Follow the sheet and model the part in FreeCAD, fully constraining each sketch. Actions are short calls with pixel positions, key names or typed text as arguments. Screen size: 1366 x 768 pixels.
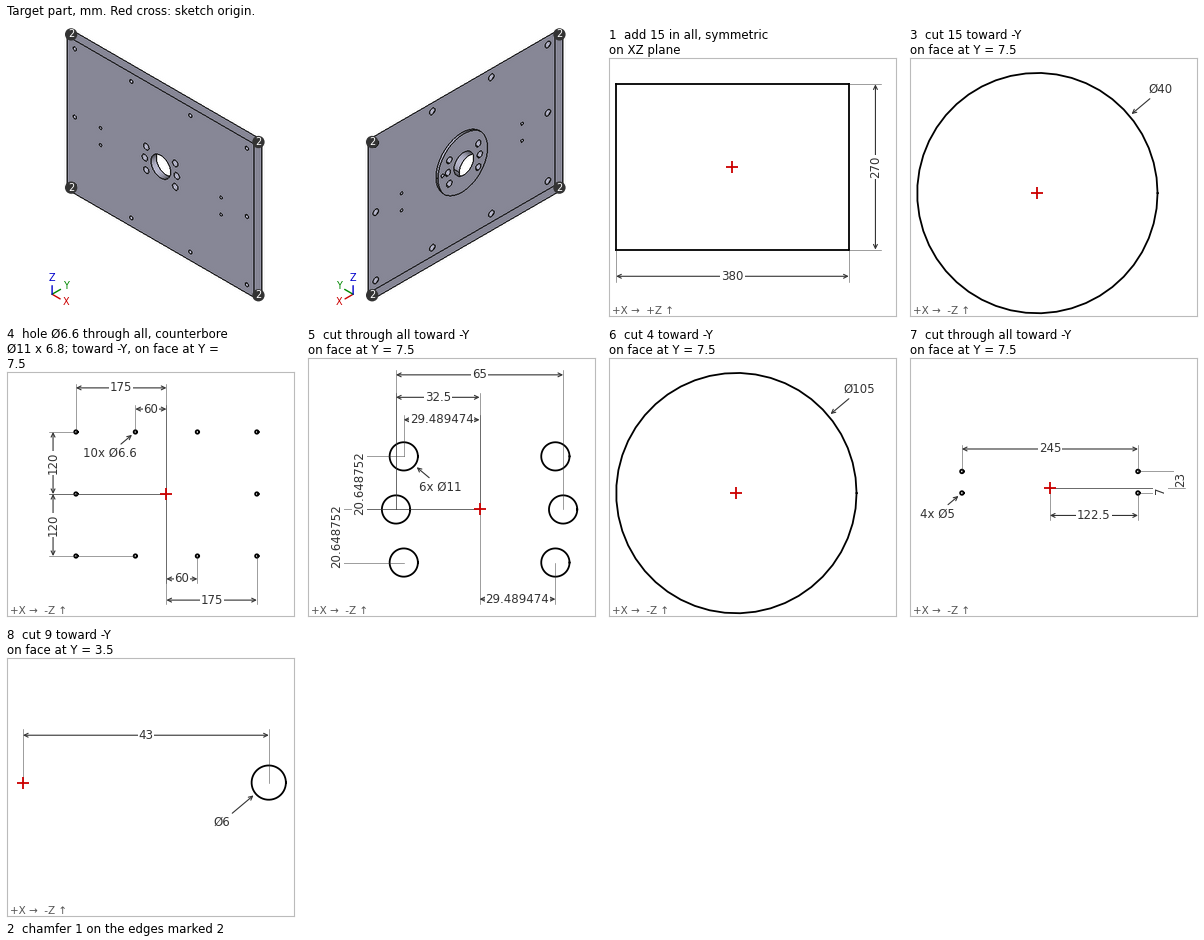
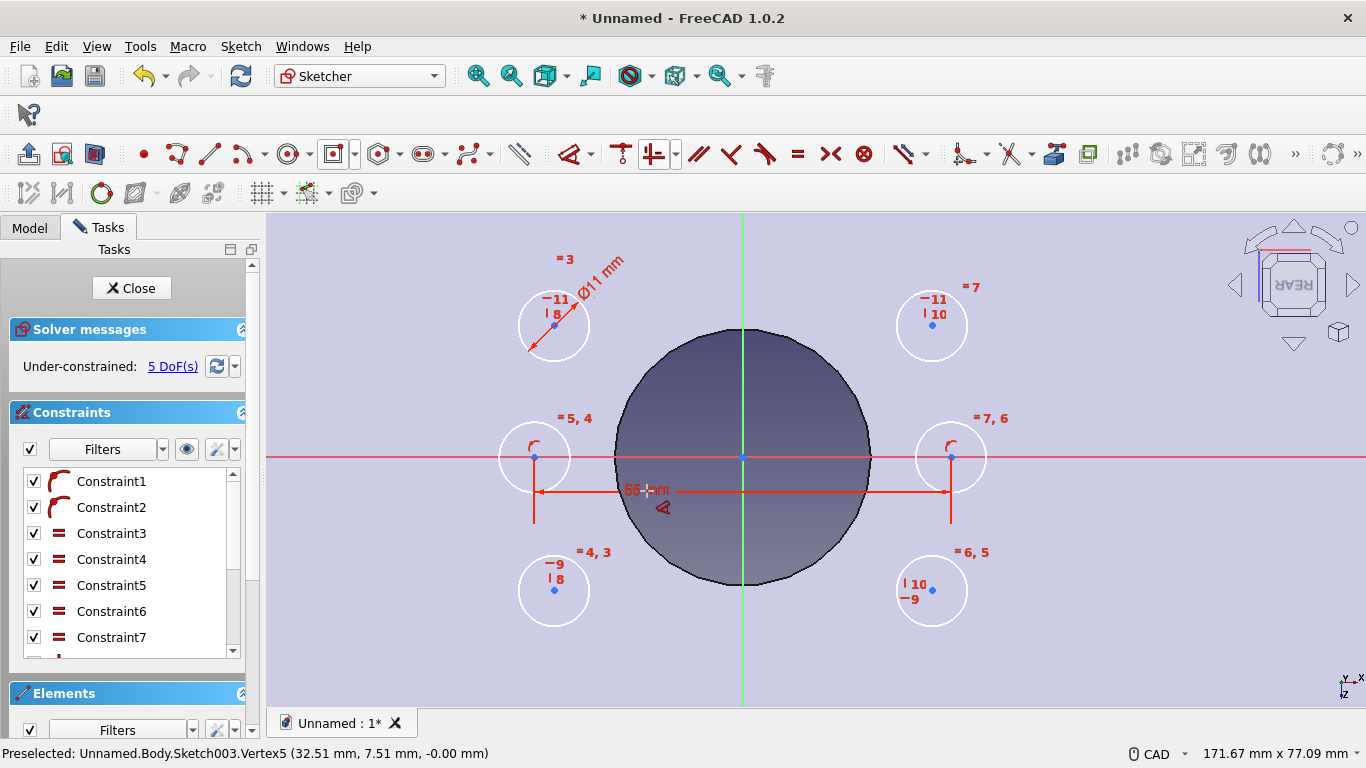
click(534, 457)
click(639, 423)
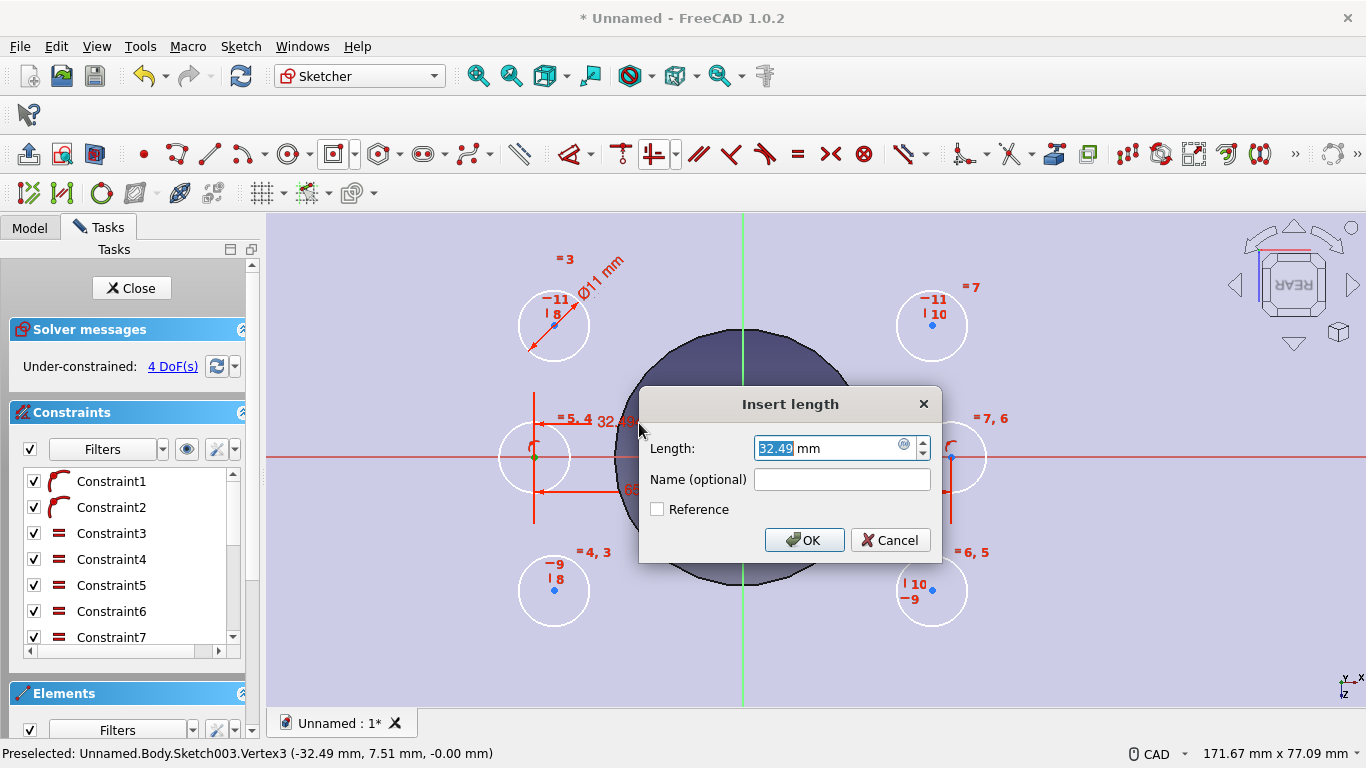
text(32.5)
key(Return)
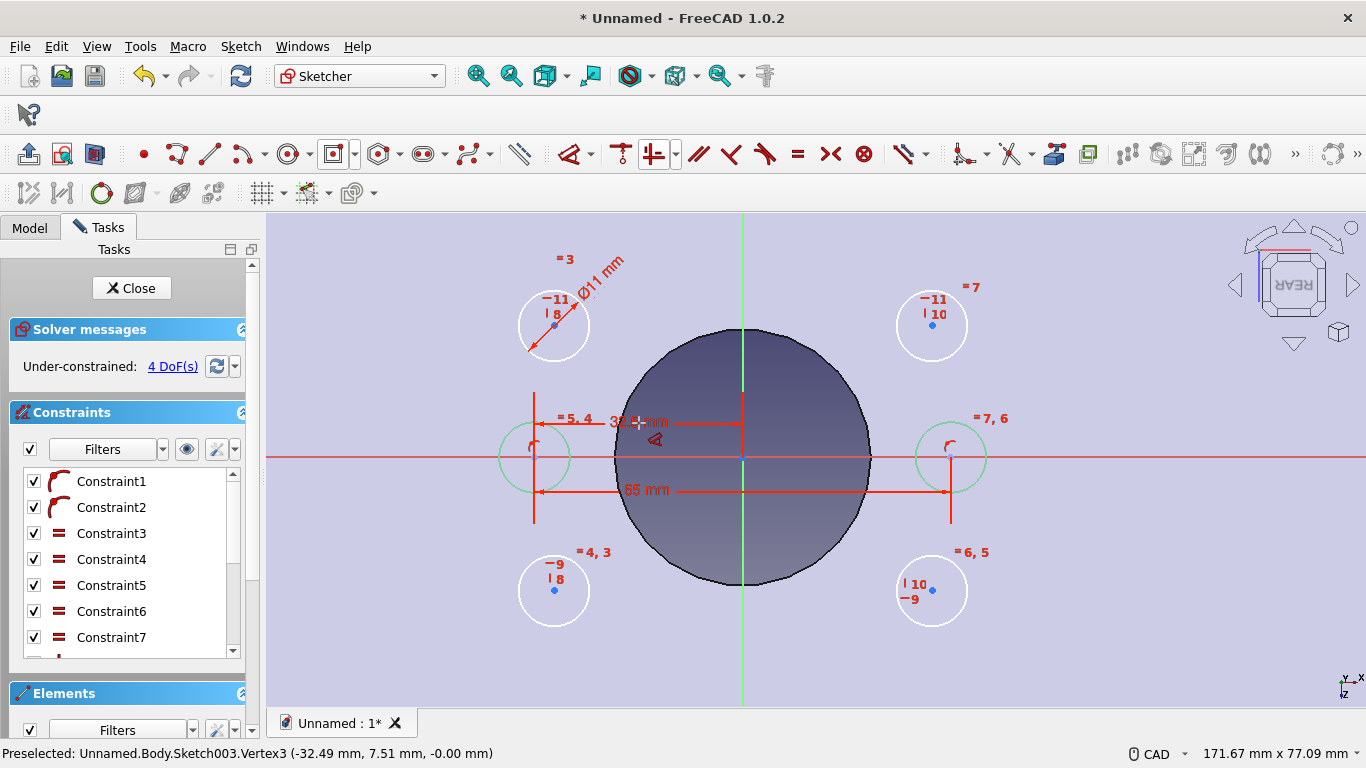
click(554, 326)
click(692, 292)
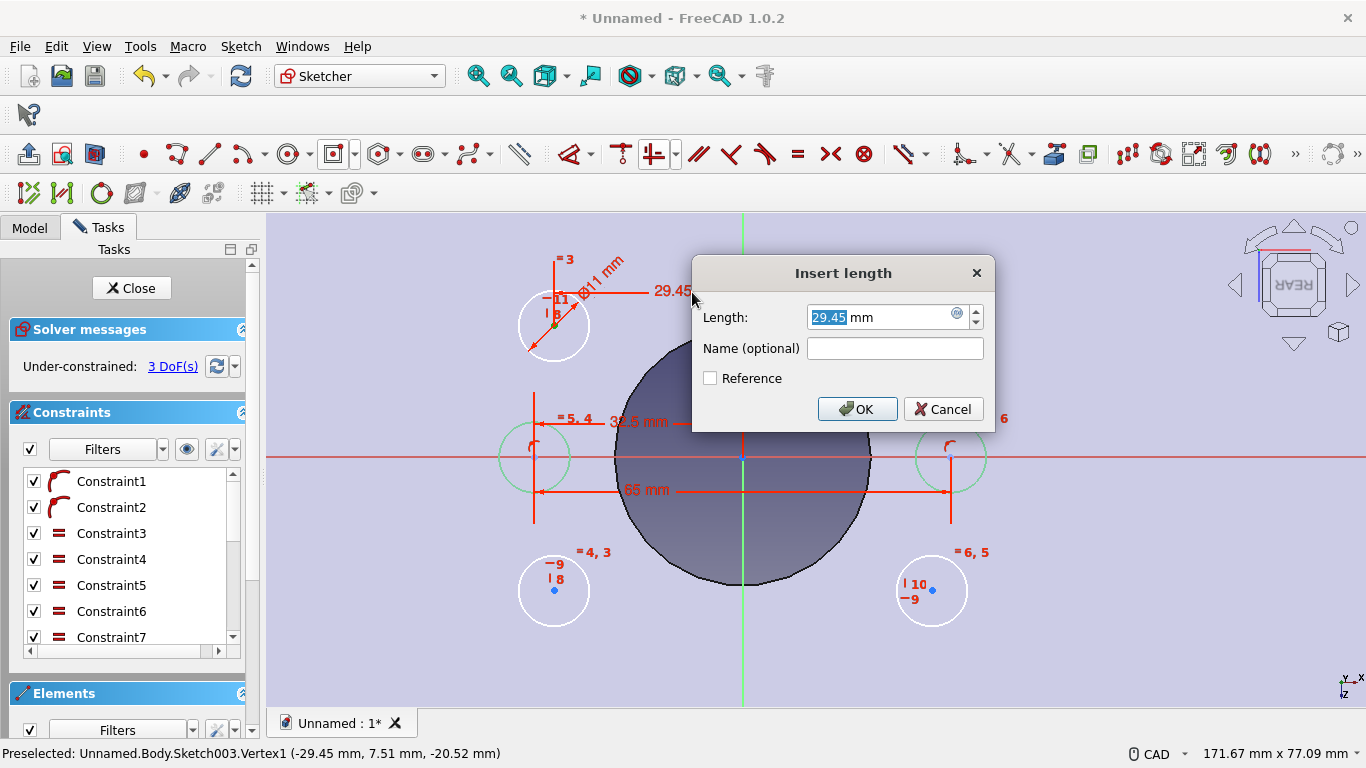
text(29.489474)
key(Return)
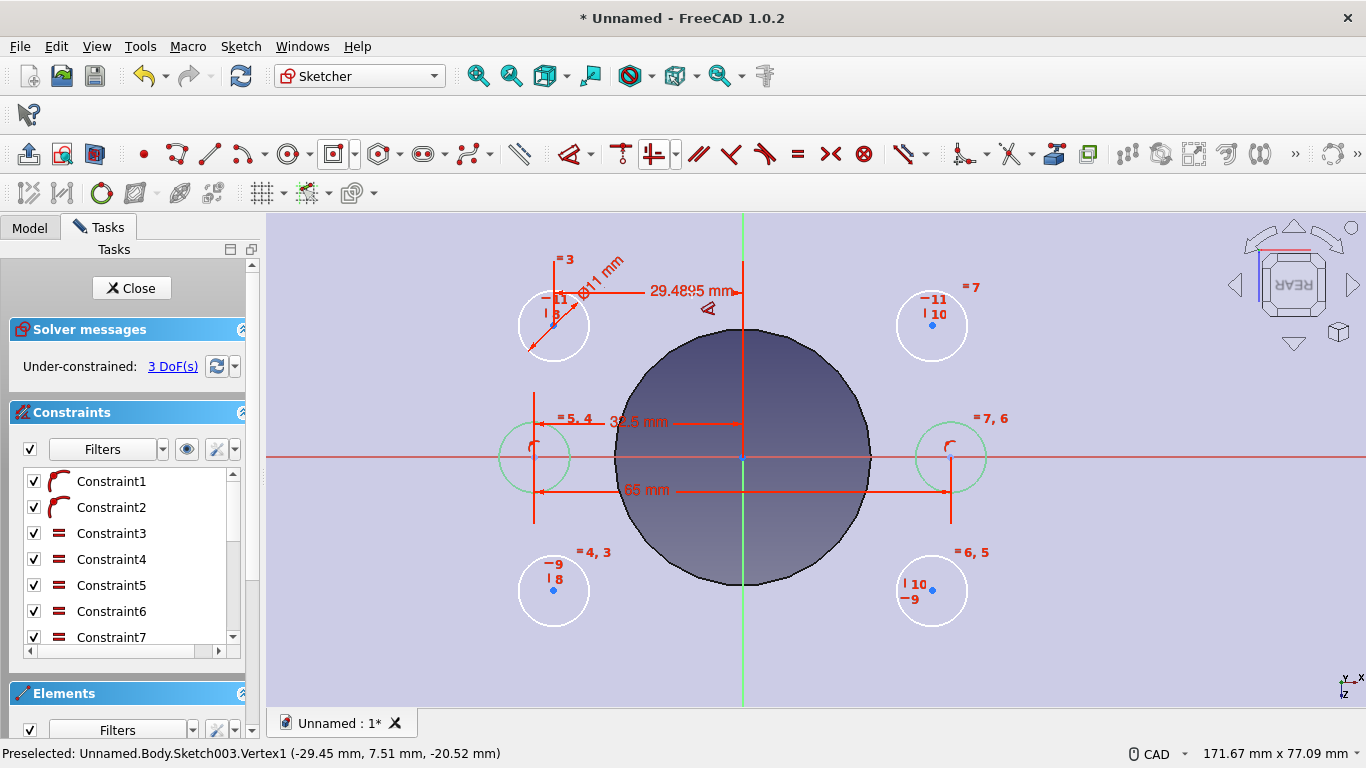
click(554, 326)
click(520, 392)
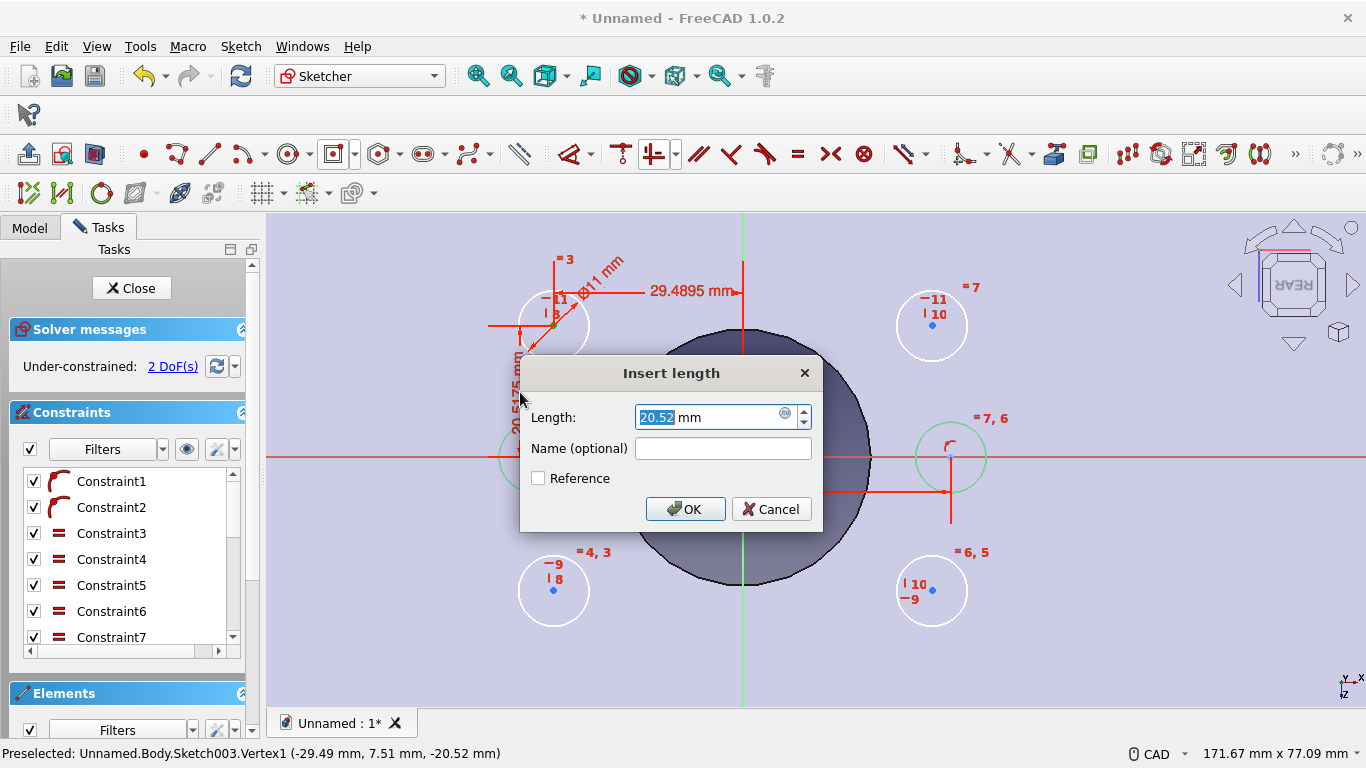
text(20.648752)
key(Return)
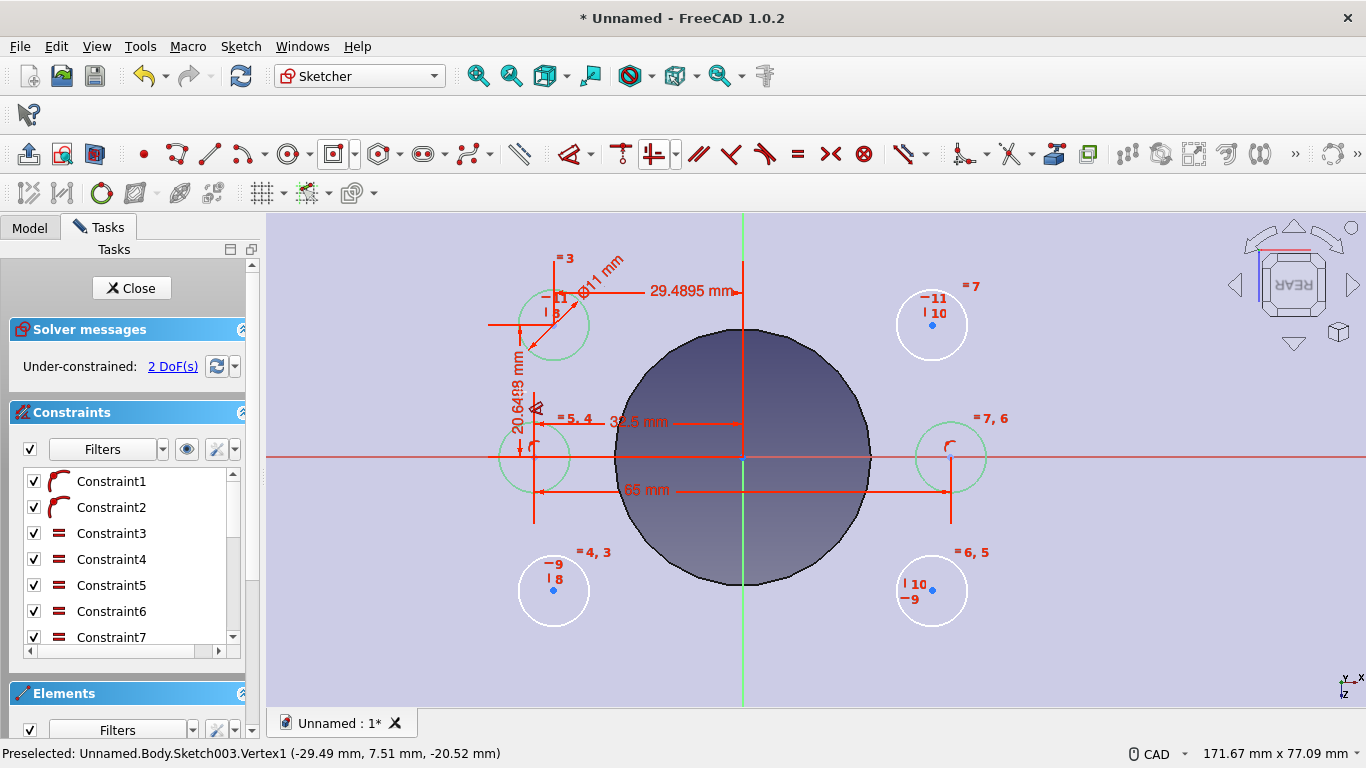
click(554, 591)
click(520, 524)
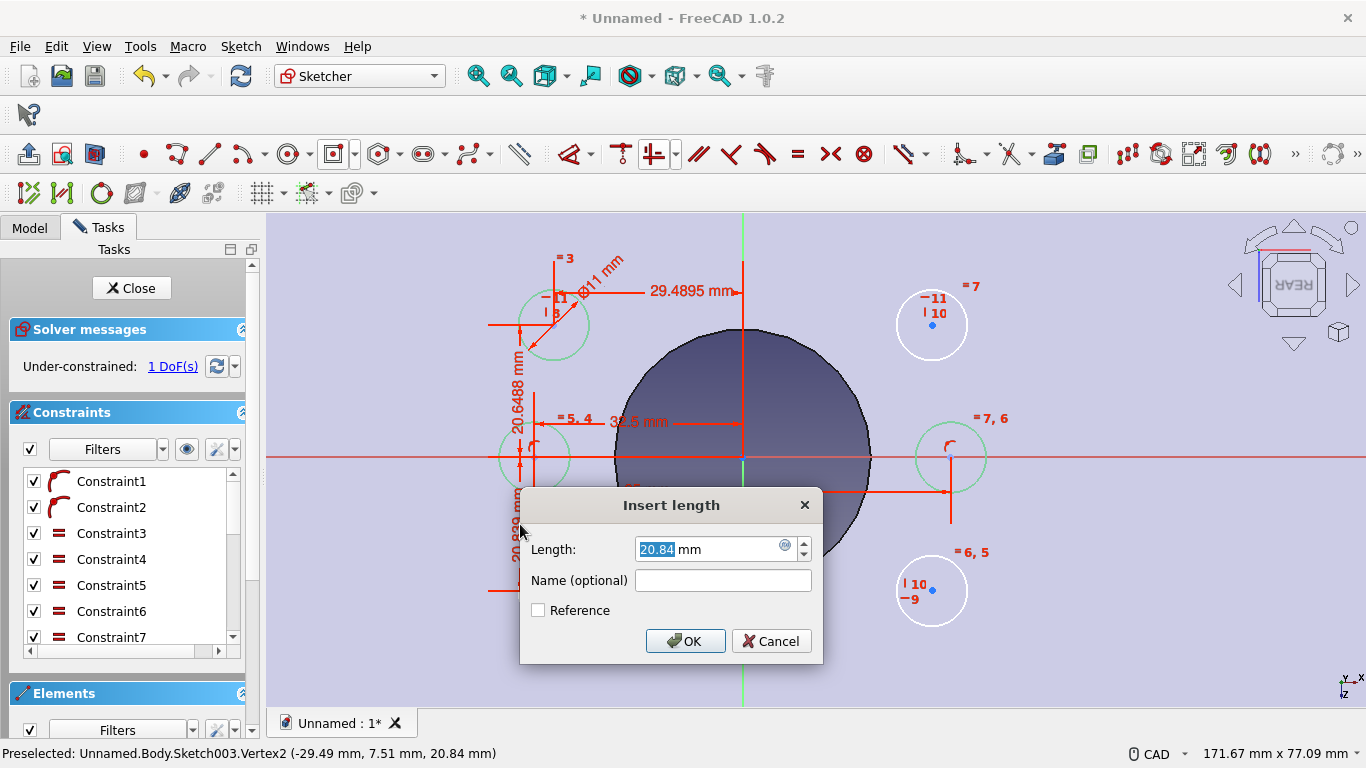
text(20.648752)
key(Return)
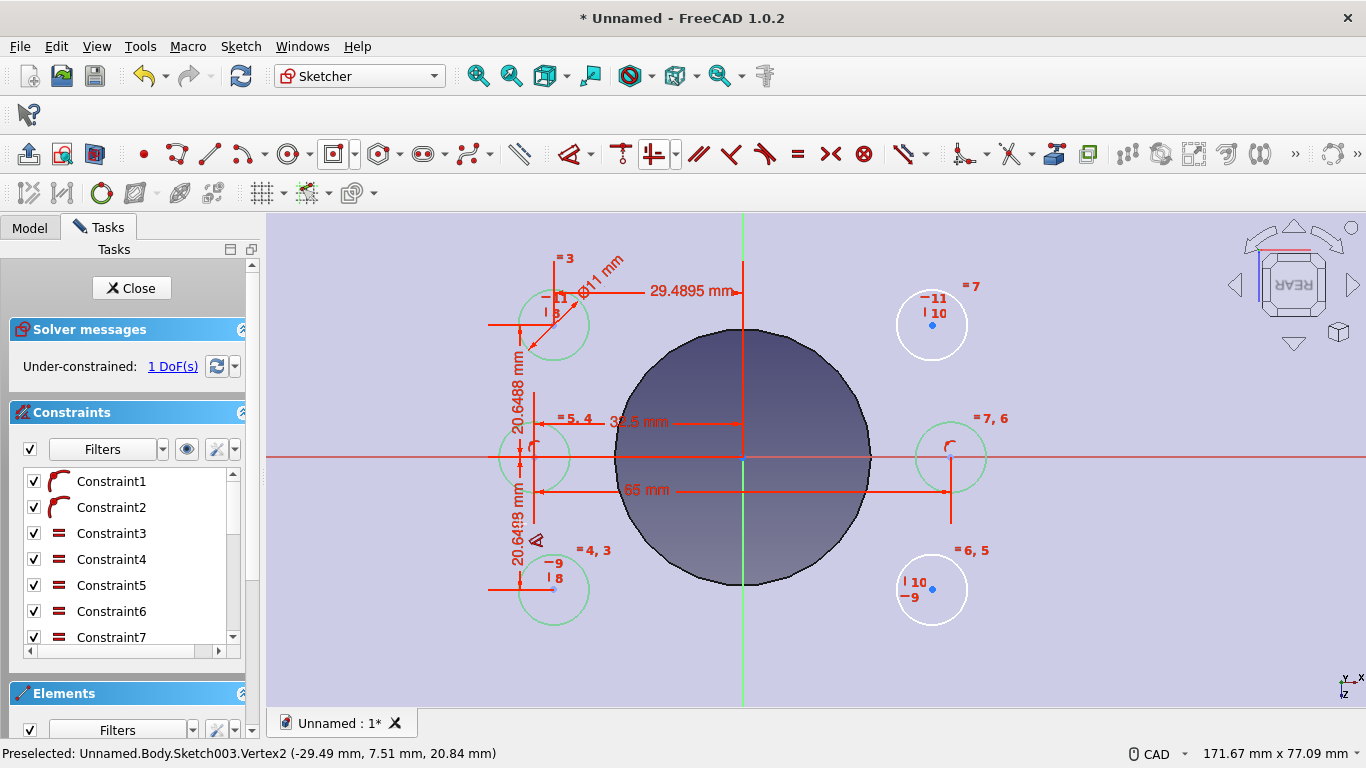
click(932, 590)
click(837, 624)